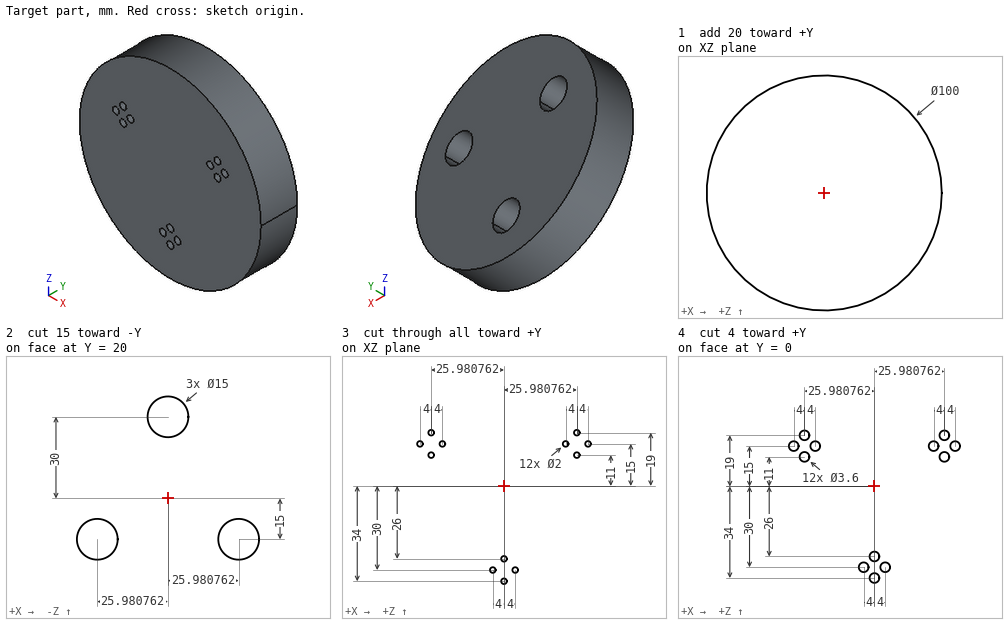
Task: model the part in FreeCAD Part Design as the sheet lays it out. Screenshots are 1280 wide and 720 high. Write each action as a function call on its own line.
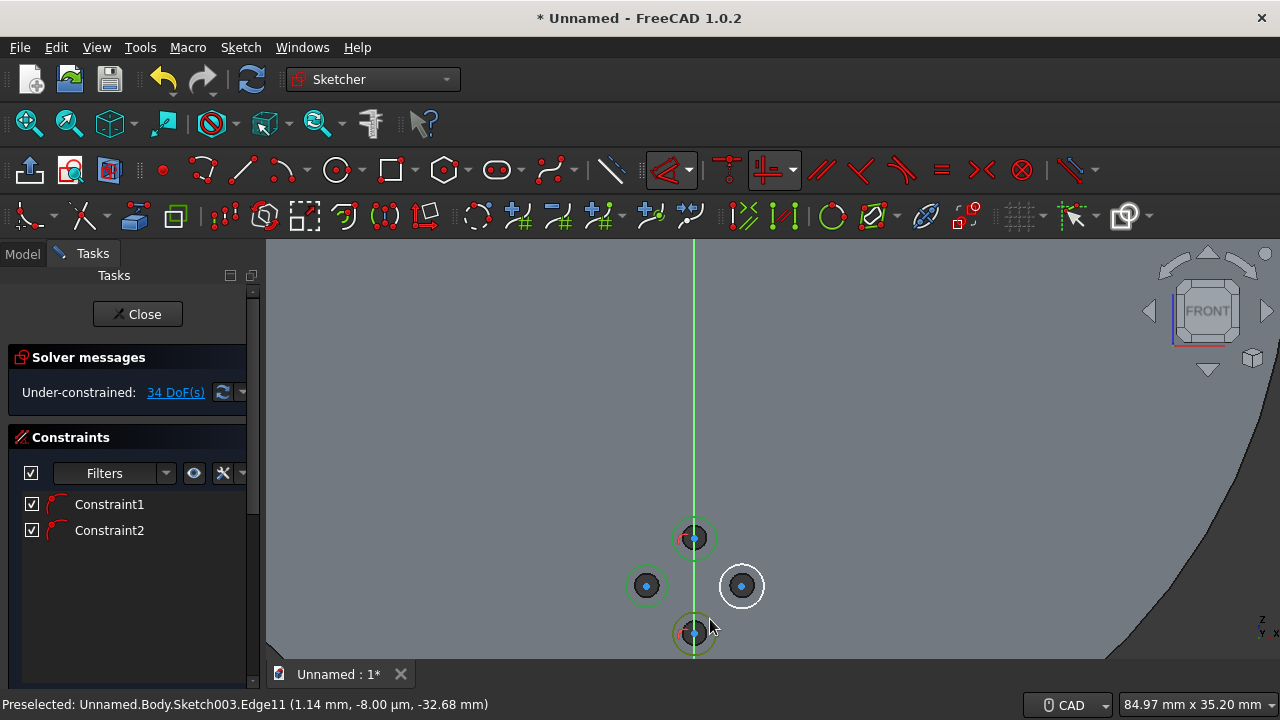
click(757, 571)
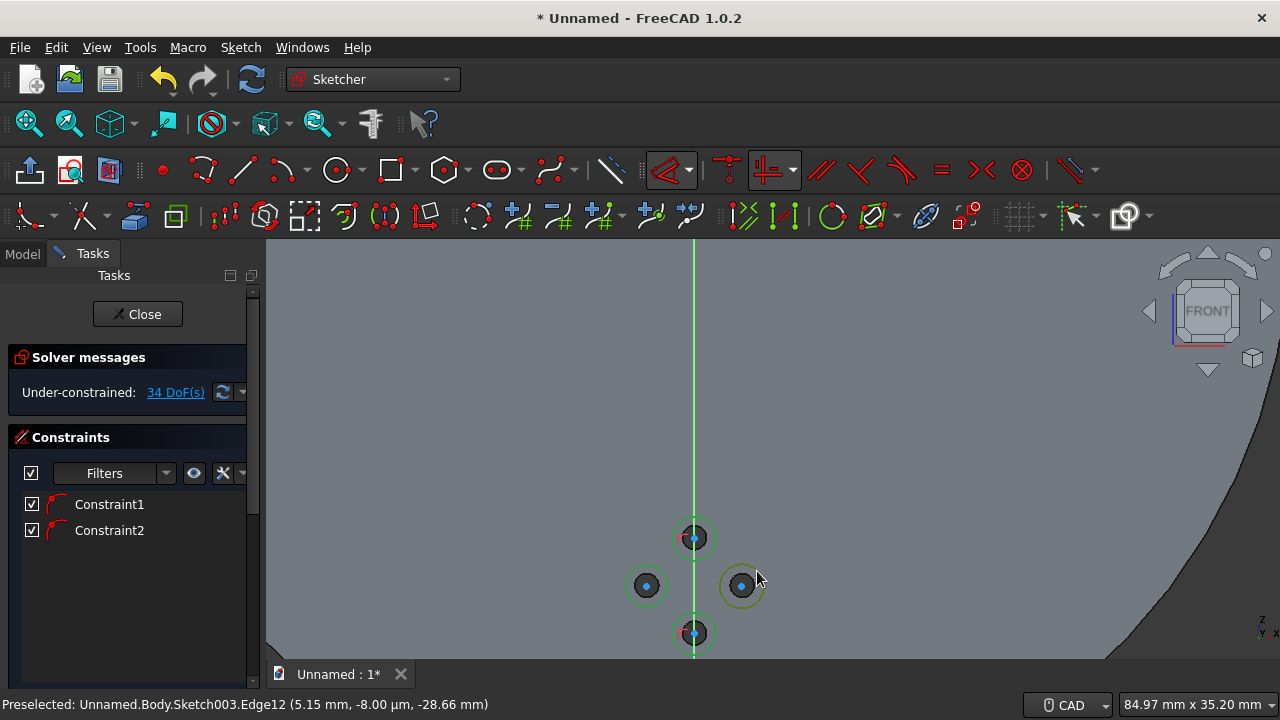
click(942, 170)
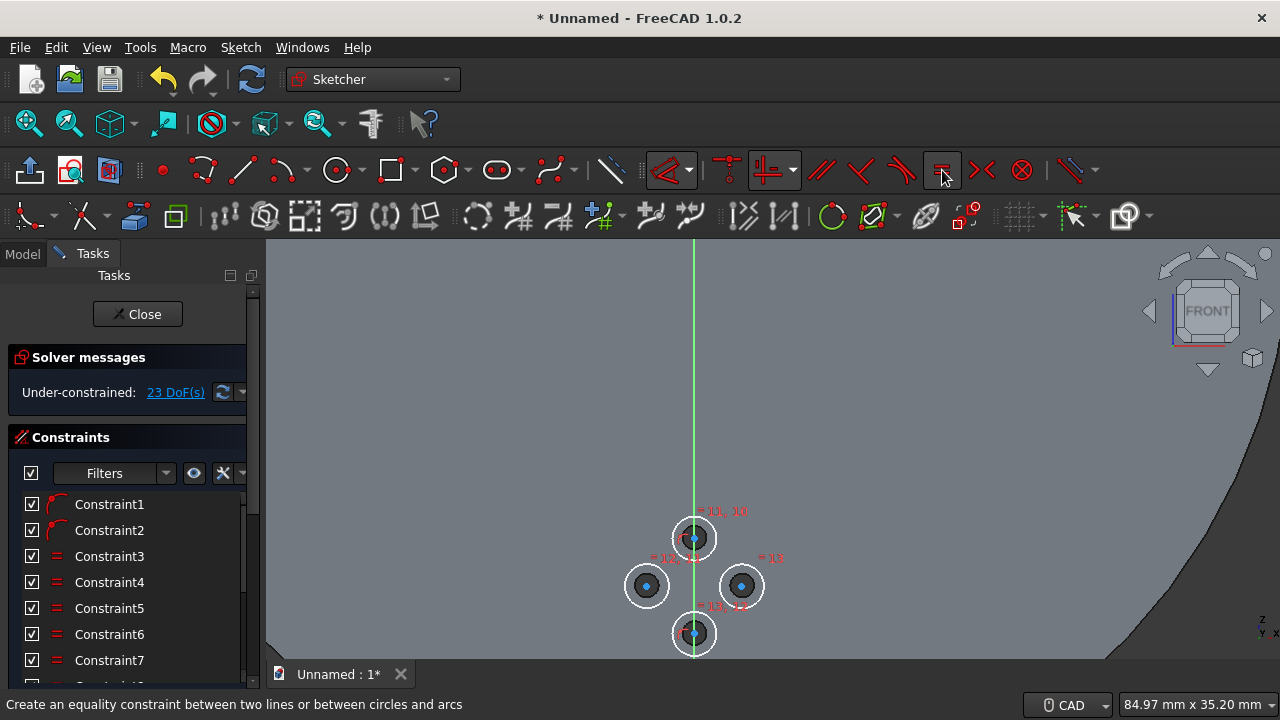
scroll(710, 526, down, 5)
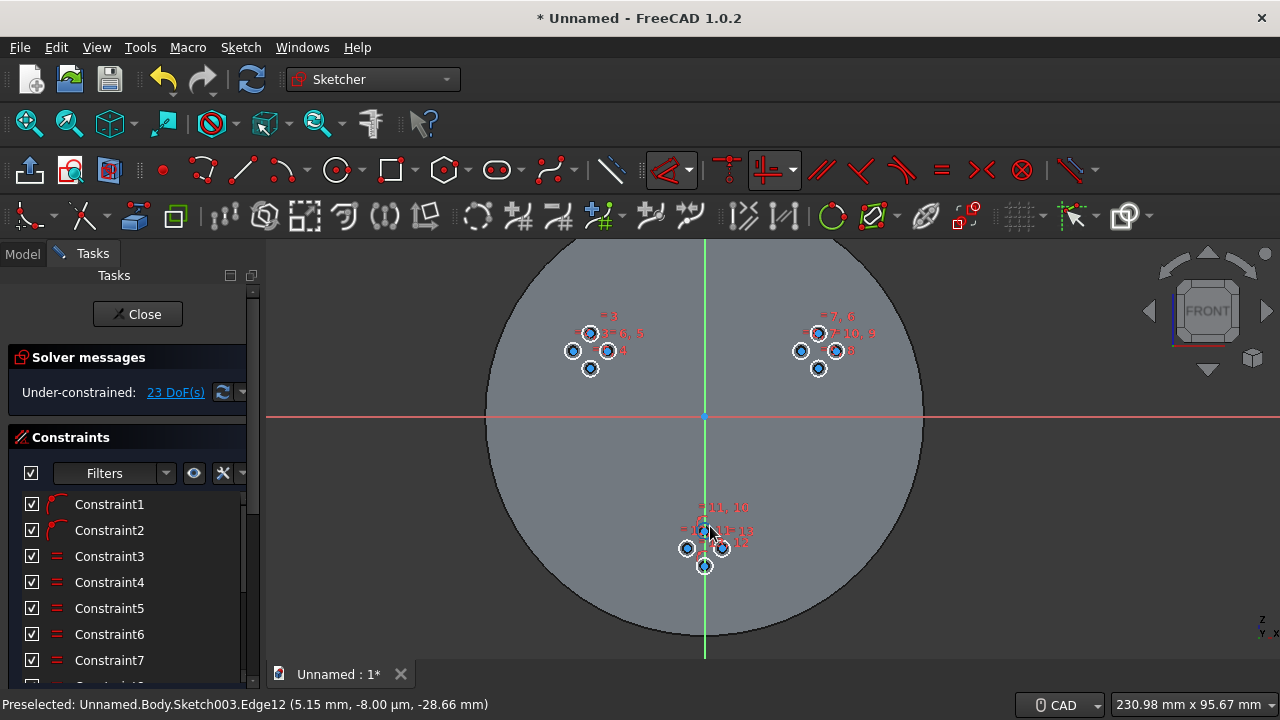
click(590, 334)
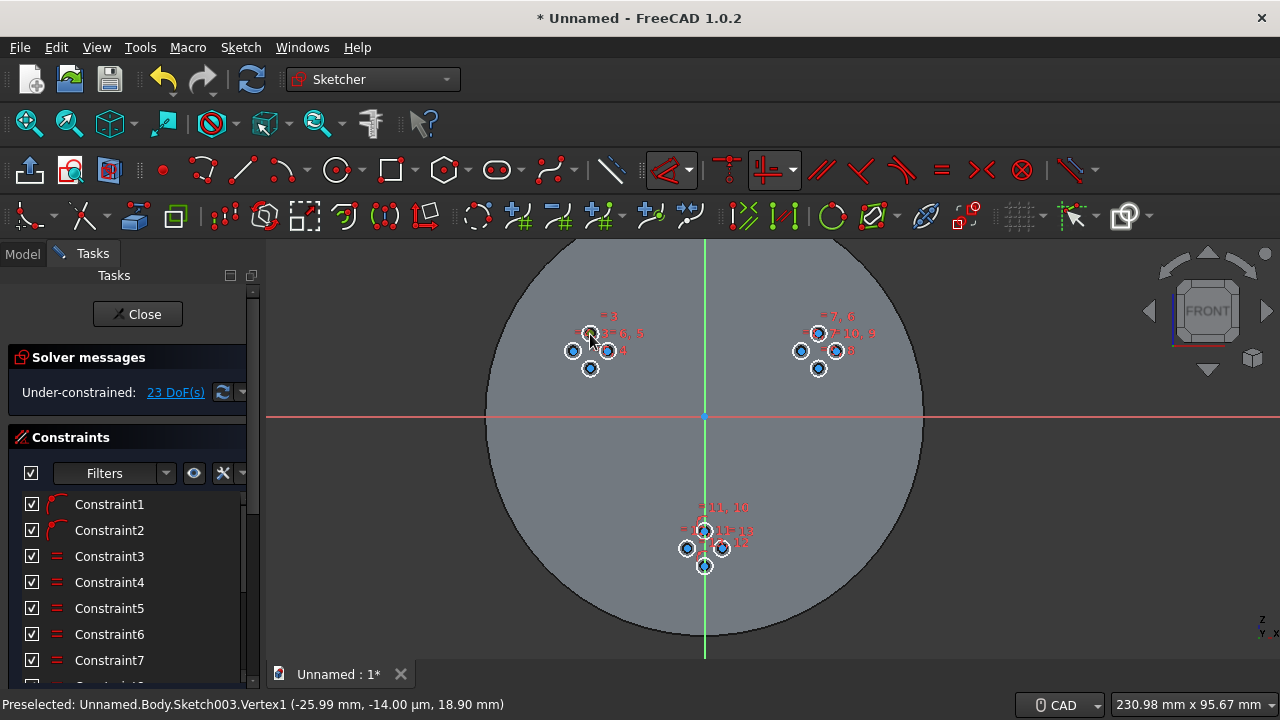
click(590, 369)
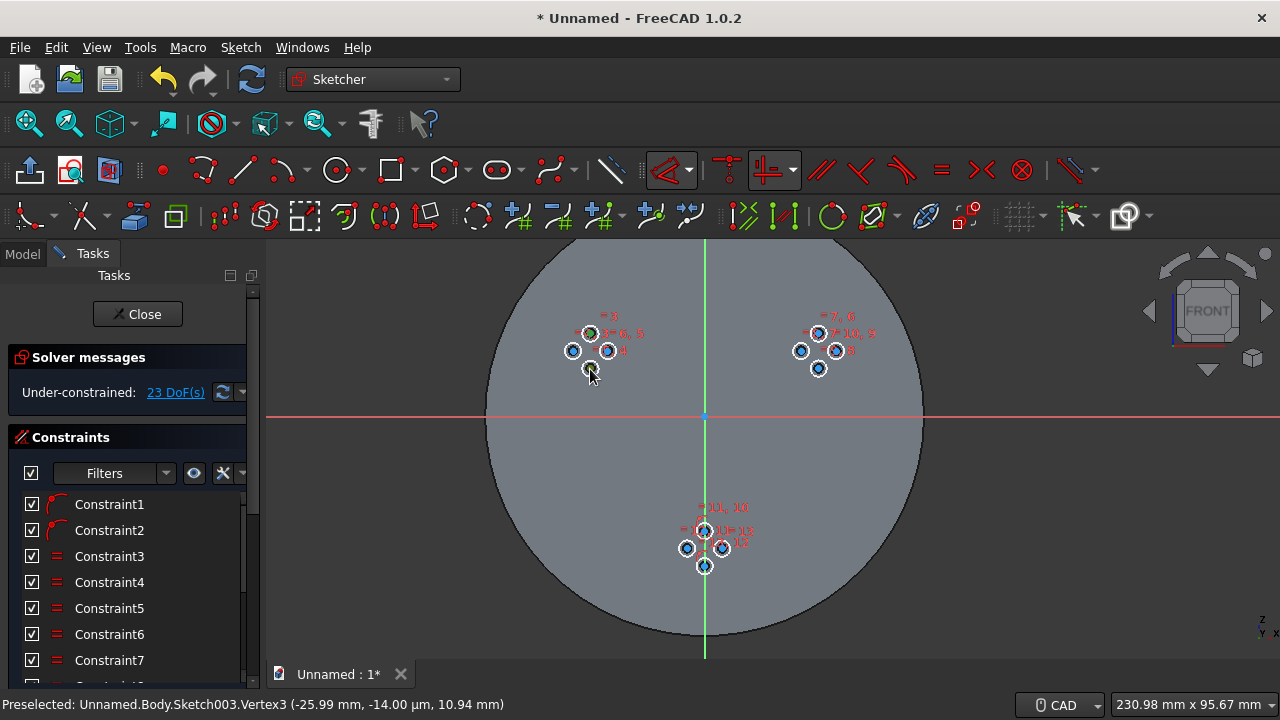
key(v)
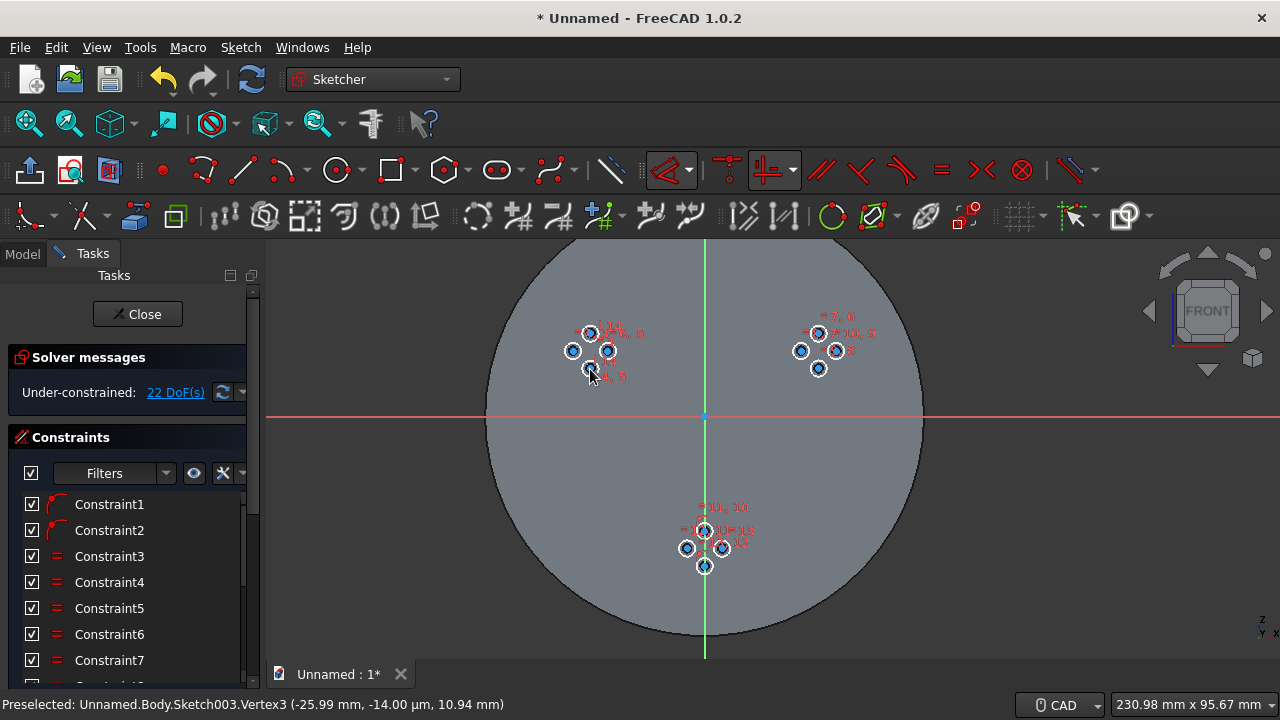
click(573, 351)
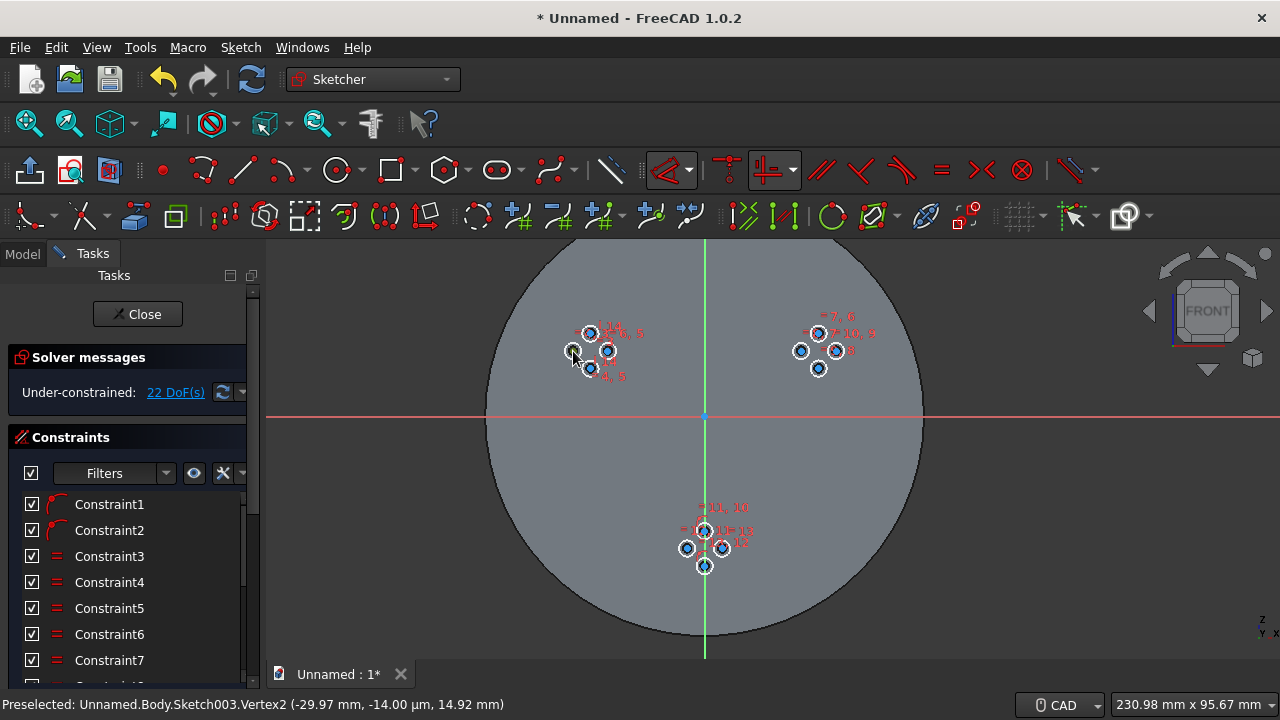
click(608, 351)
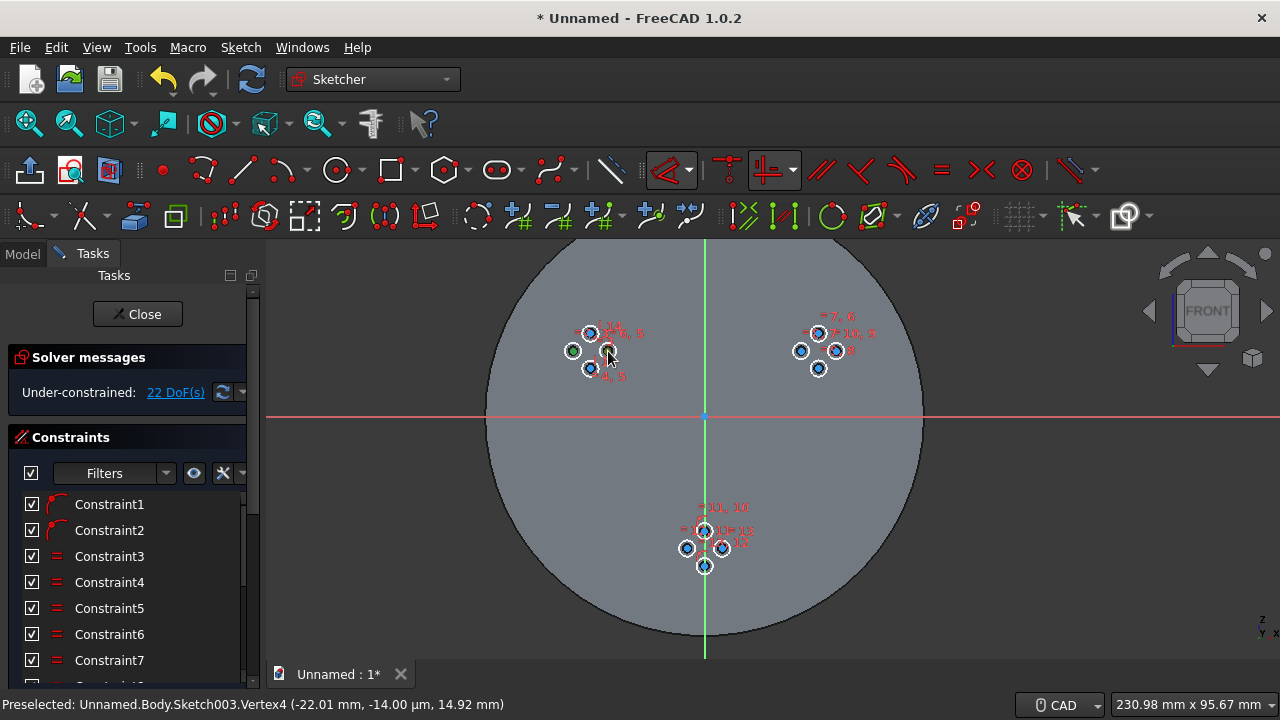
click(796, 170)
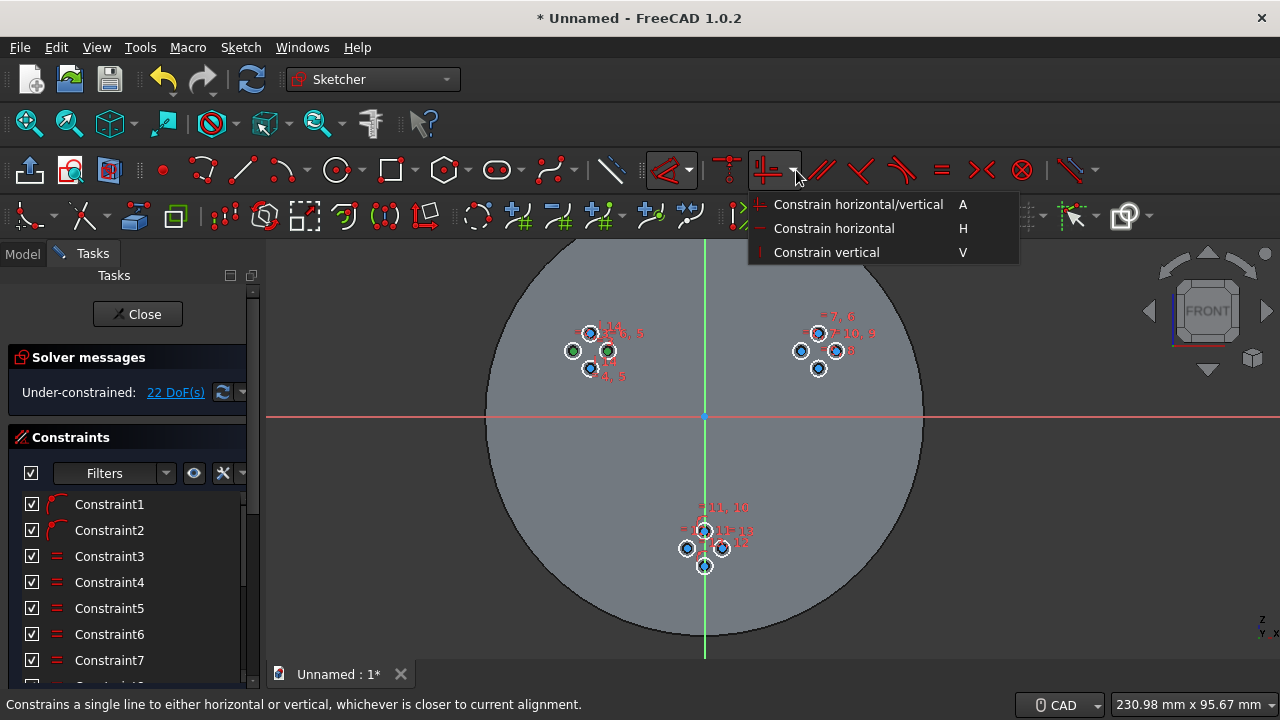
click(884, 228)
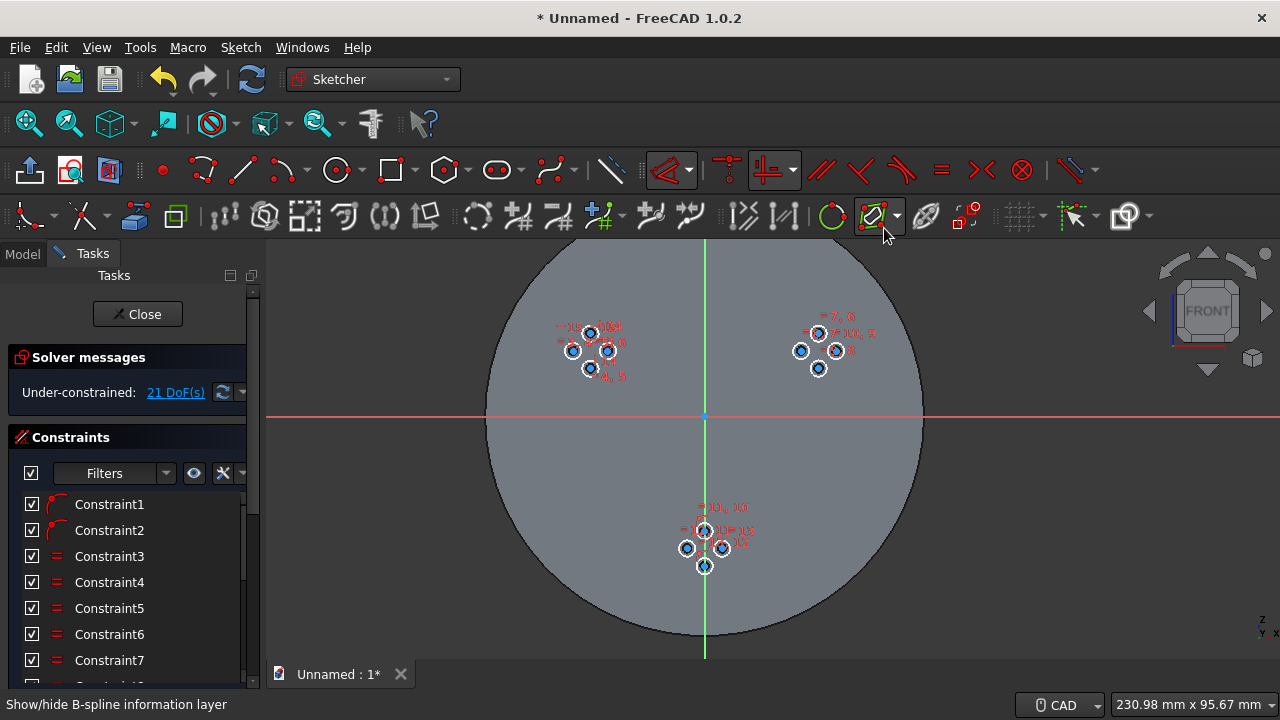
click(588, 336)